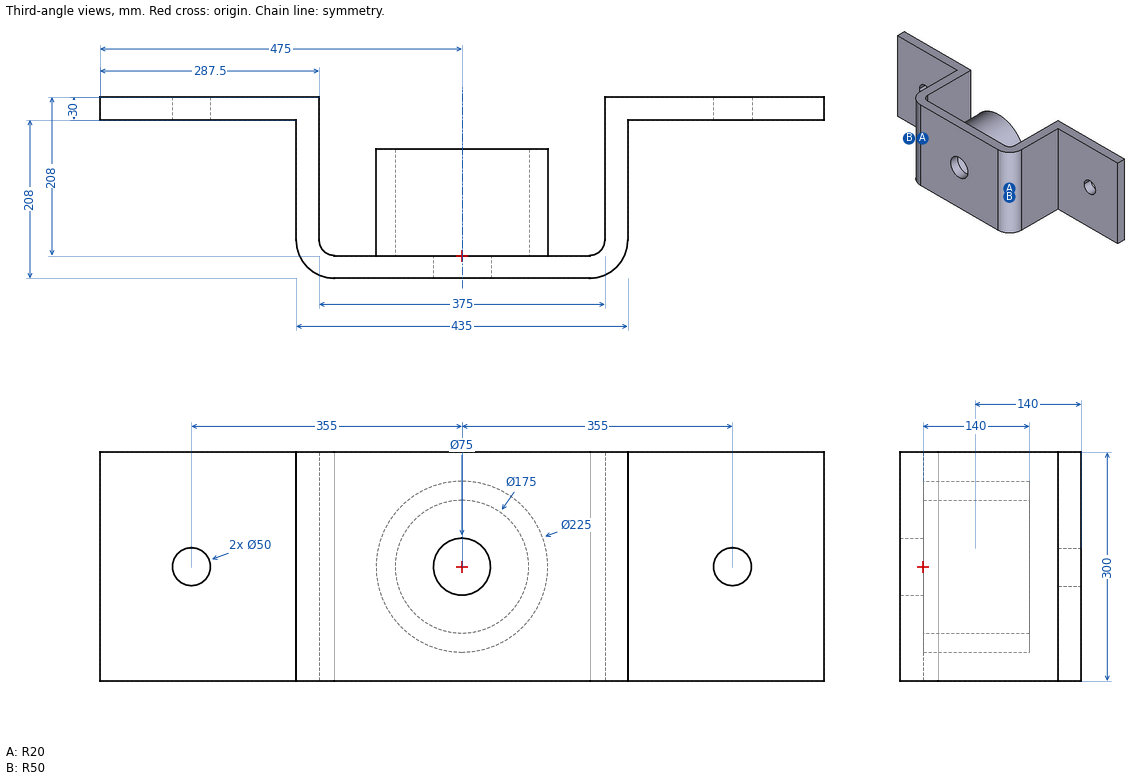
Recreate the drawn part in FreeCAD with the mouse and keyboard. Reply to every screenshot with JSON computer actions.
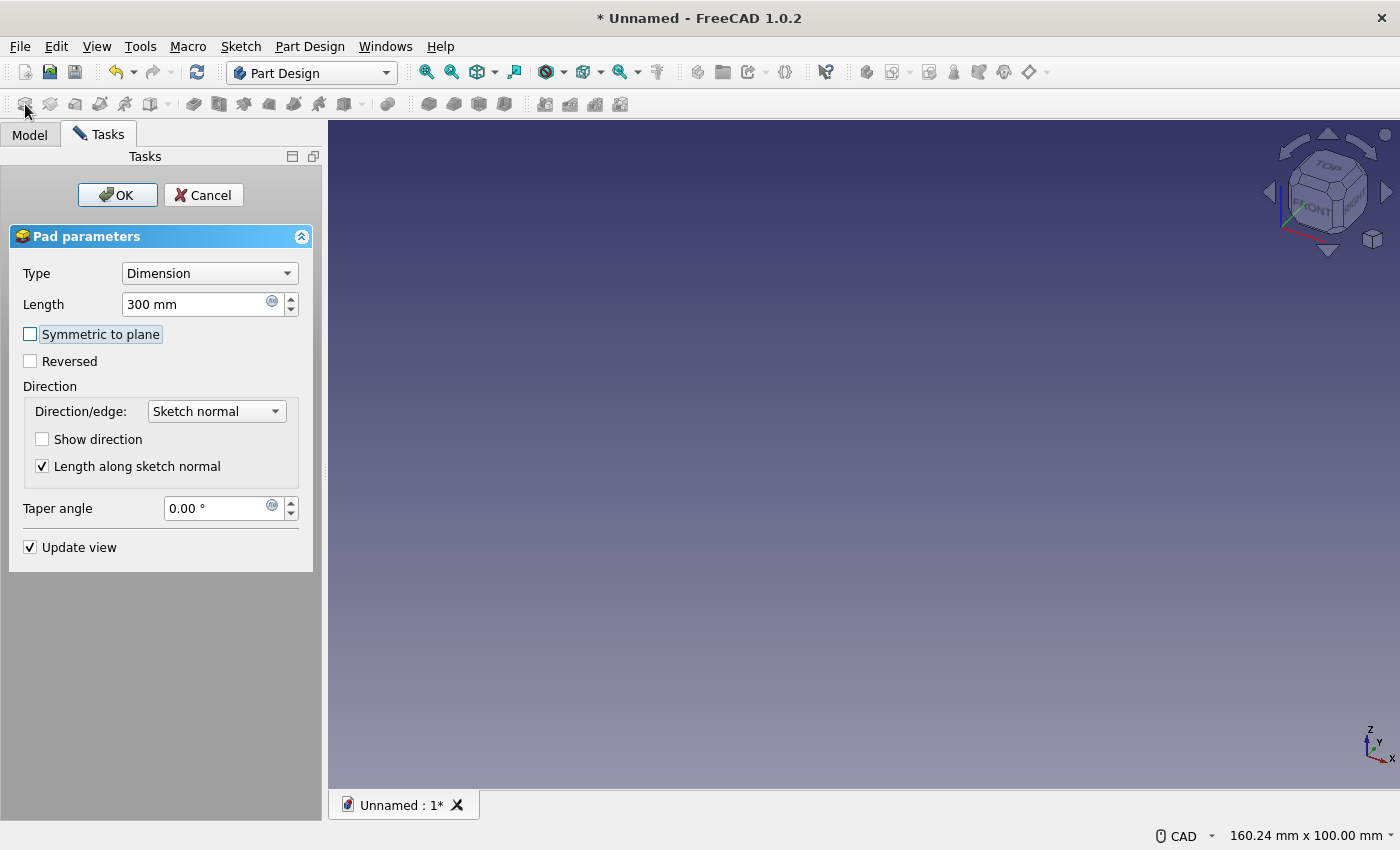
{"action": "left_click", "coordinate": [31, 334]}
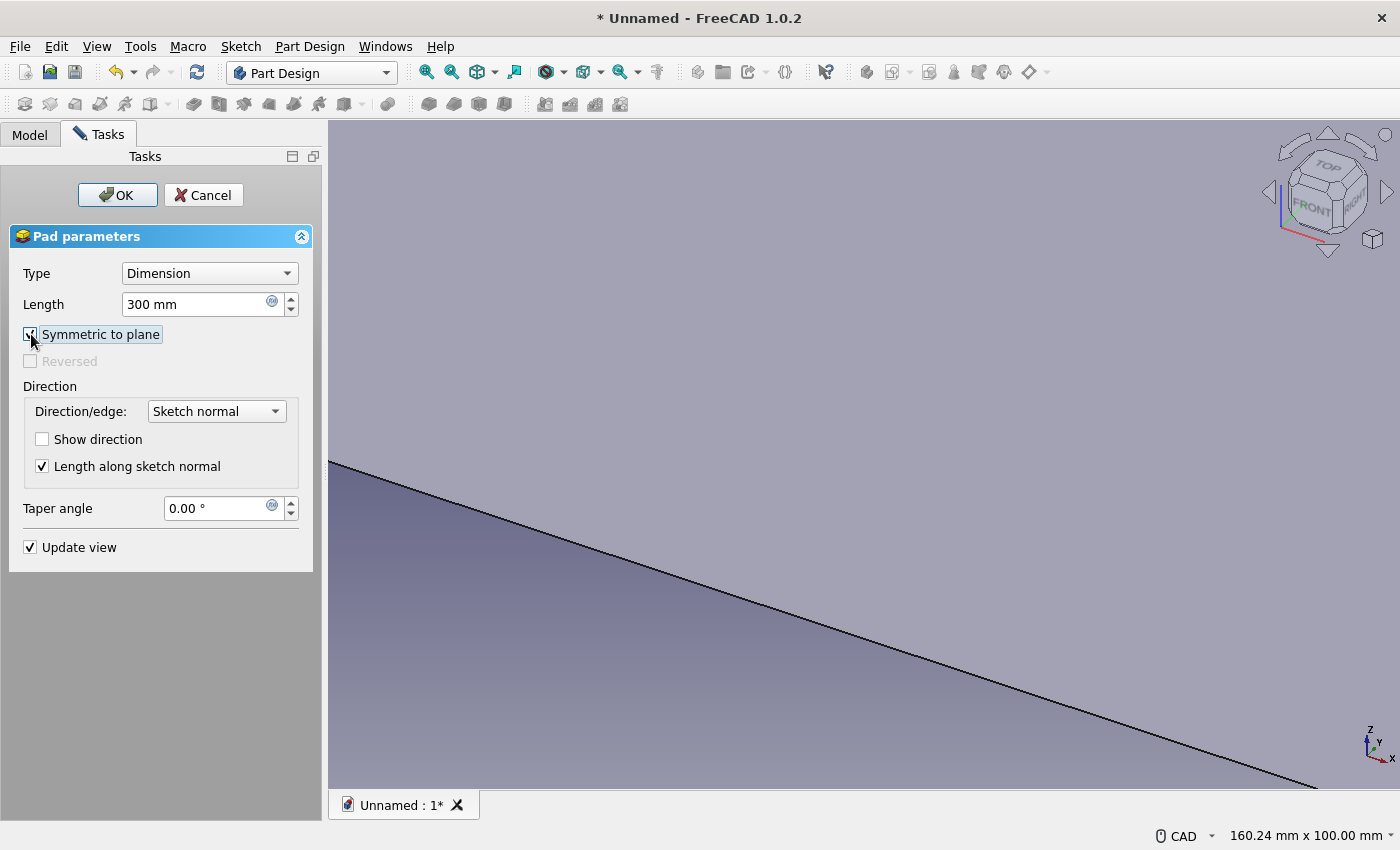
{"action": "left_click", "coordinate": [118, 195]}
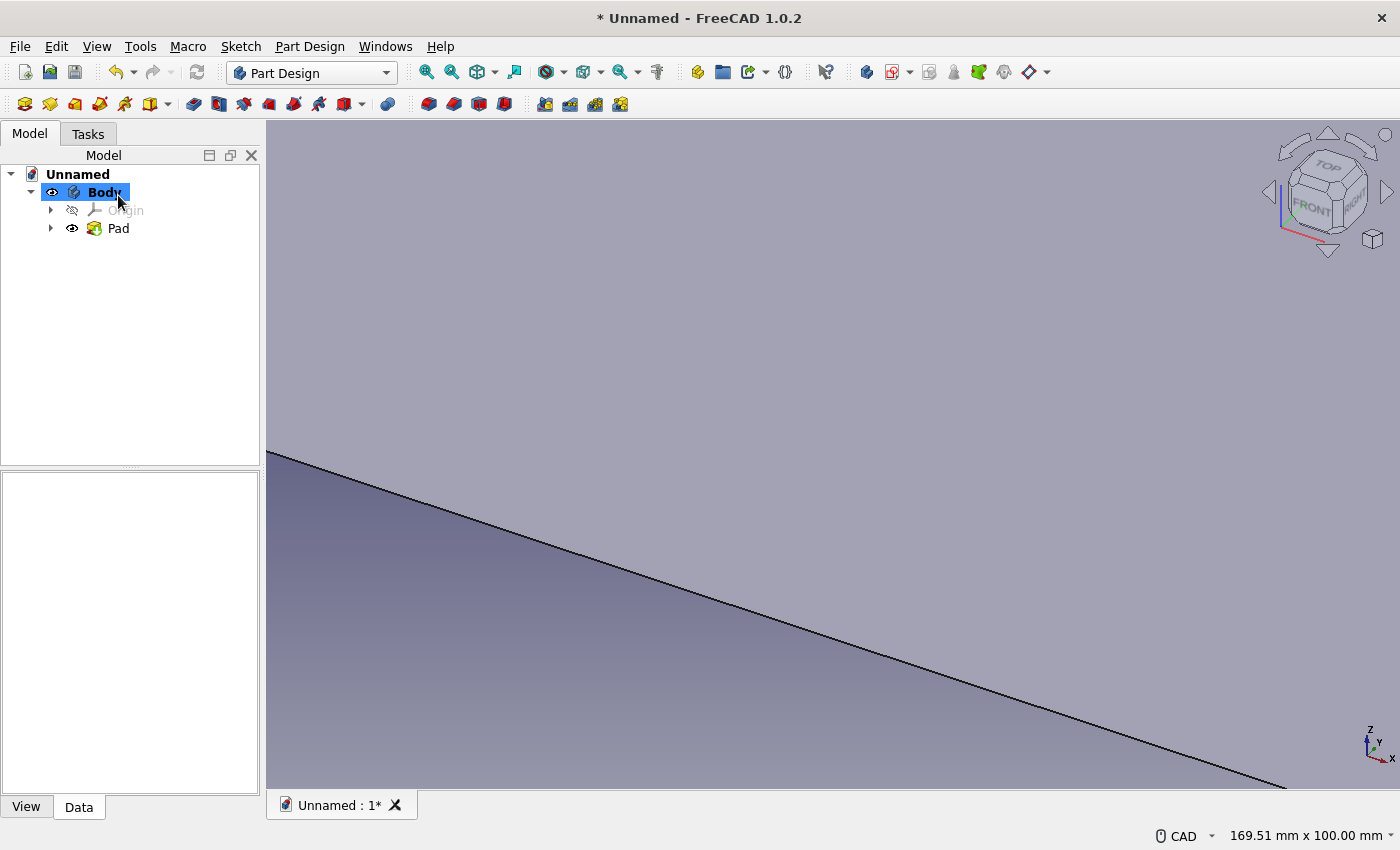
{"action": "left_click", "coordinate": [427, 72]}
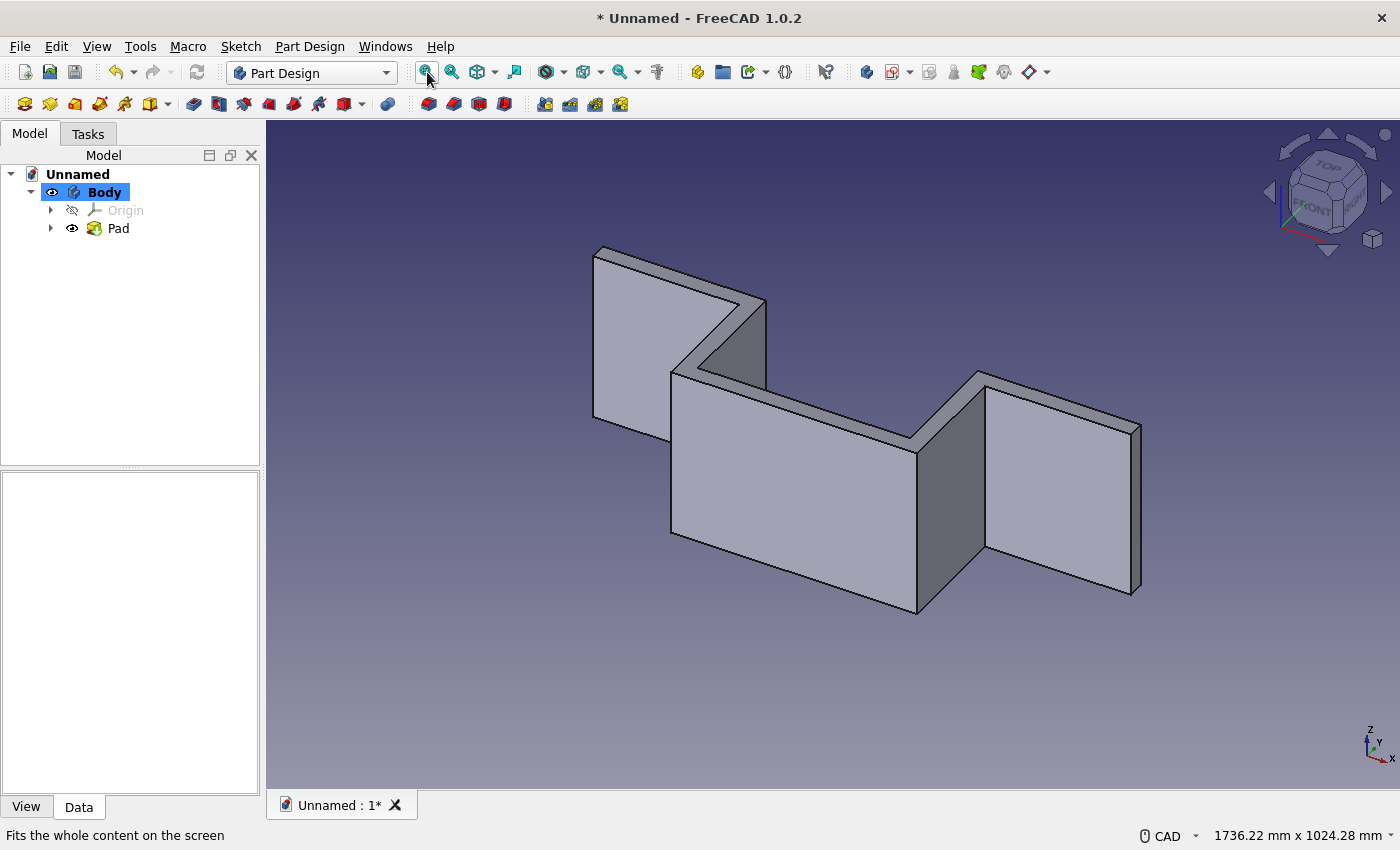
{"action": "key", "text": "4"}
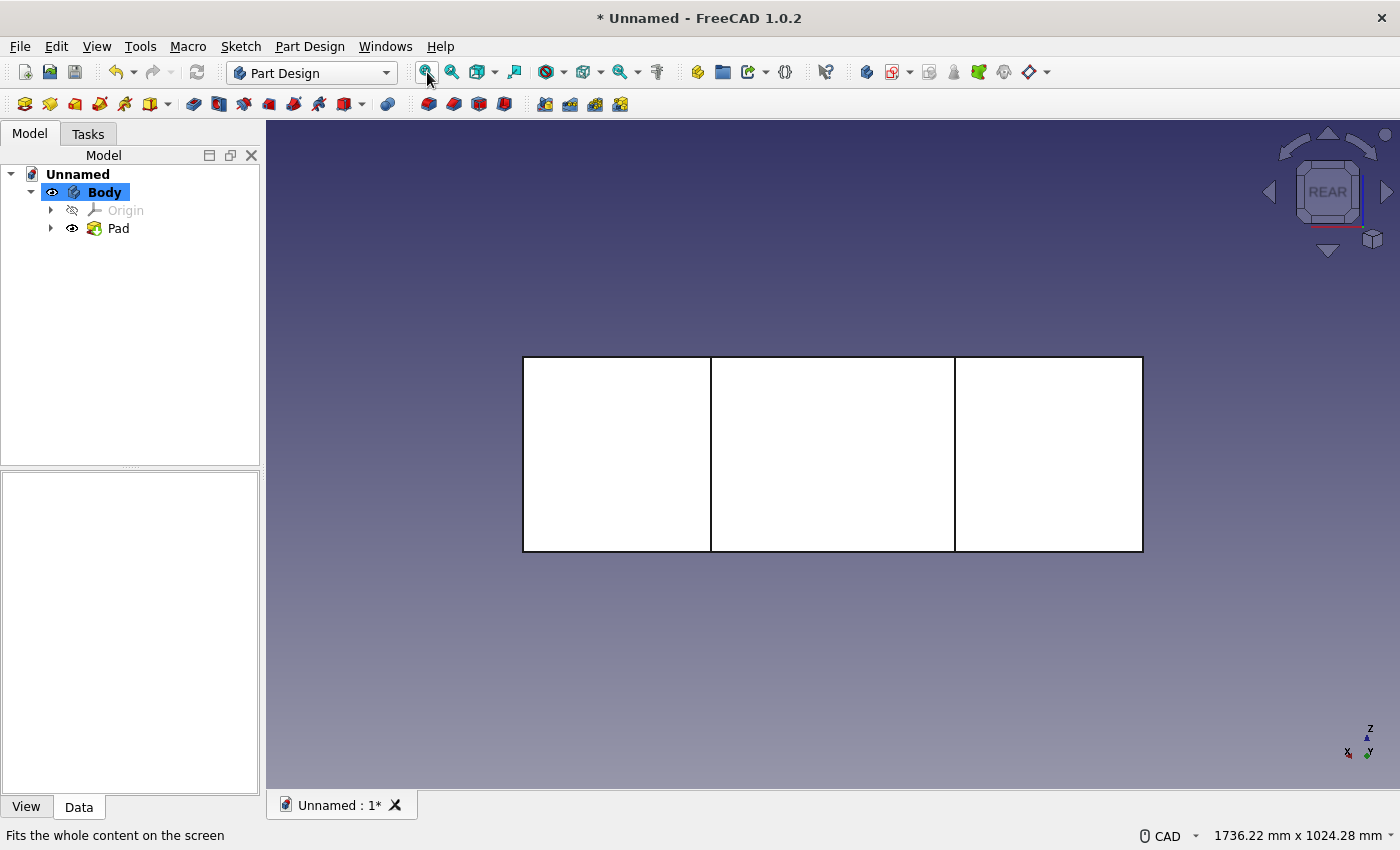
{"action": "left_click", "coordinate": [833, 453]}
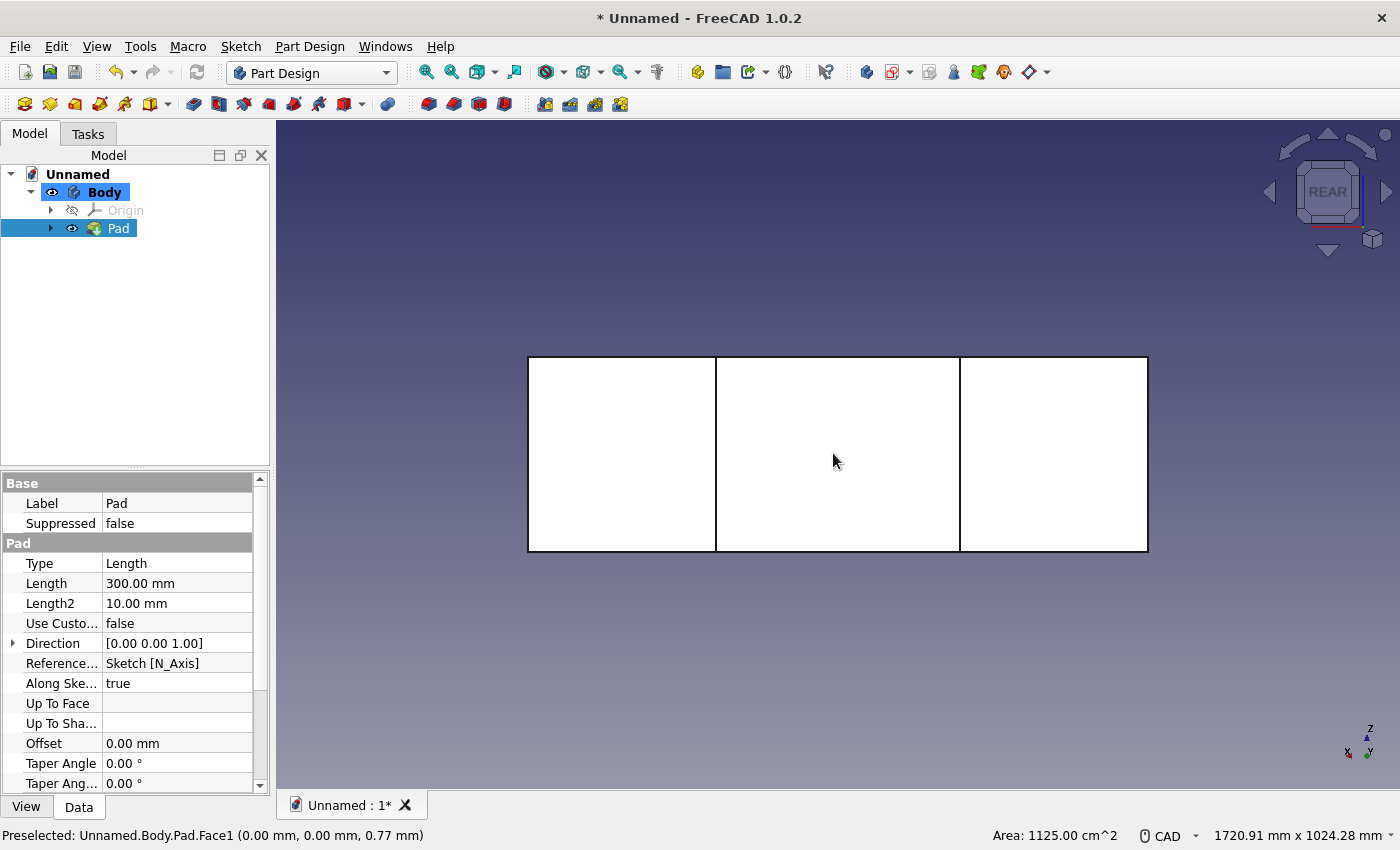
{"action": "left_click", "coordinate": [892, 72]}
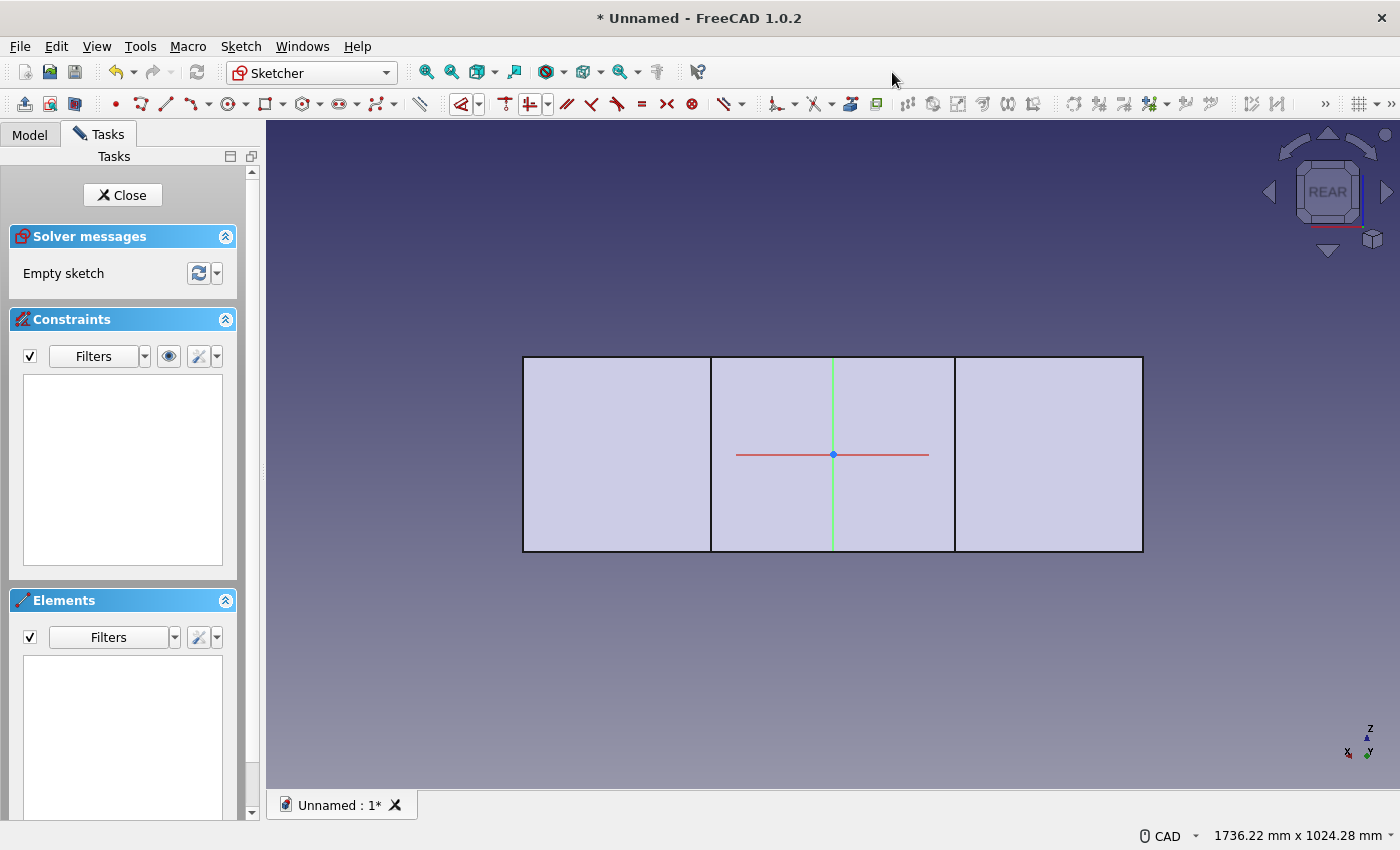
{"action": "scroll", "coordinate": [873, 454], "scroll_direction": "up", "scroll_amount": 5}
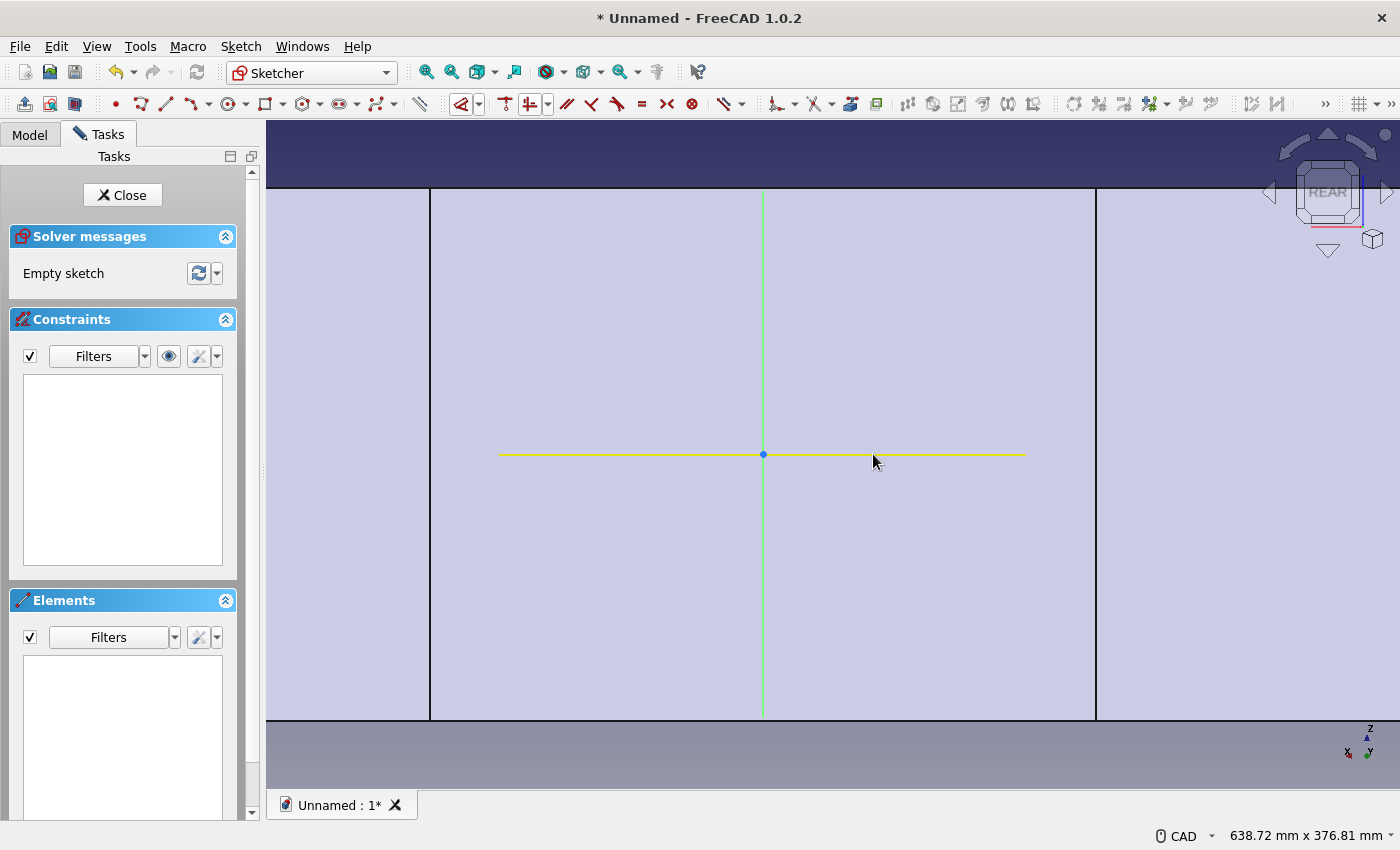
{"action": "left_click", "coordinate": [228, 104]}